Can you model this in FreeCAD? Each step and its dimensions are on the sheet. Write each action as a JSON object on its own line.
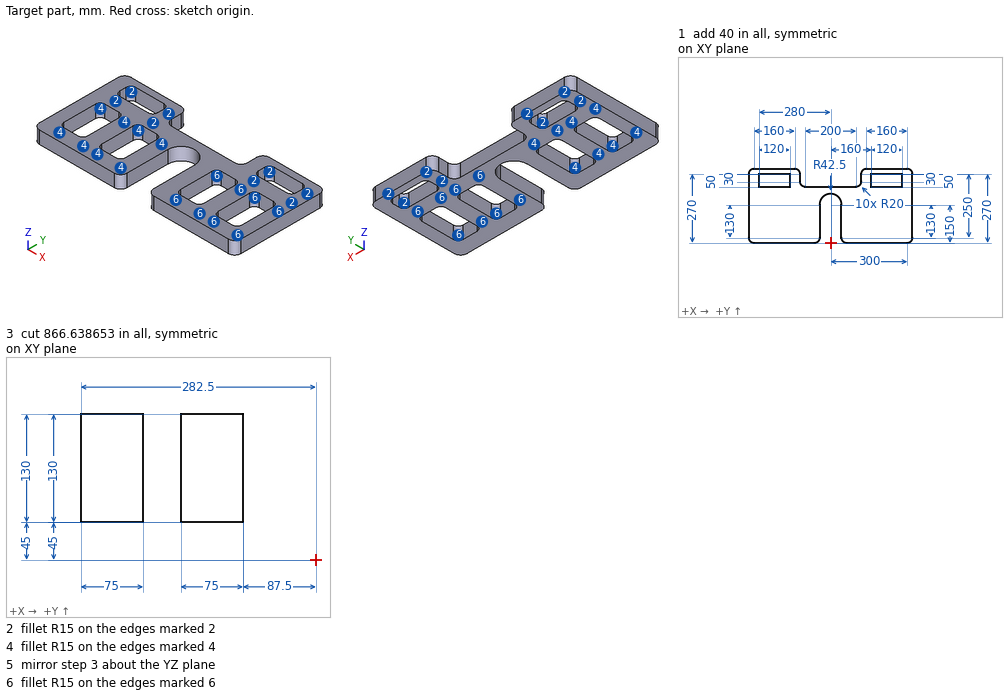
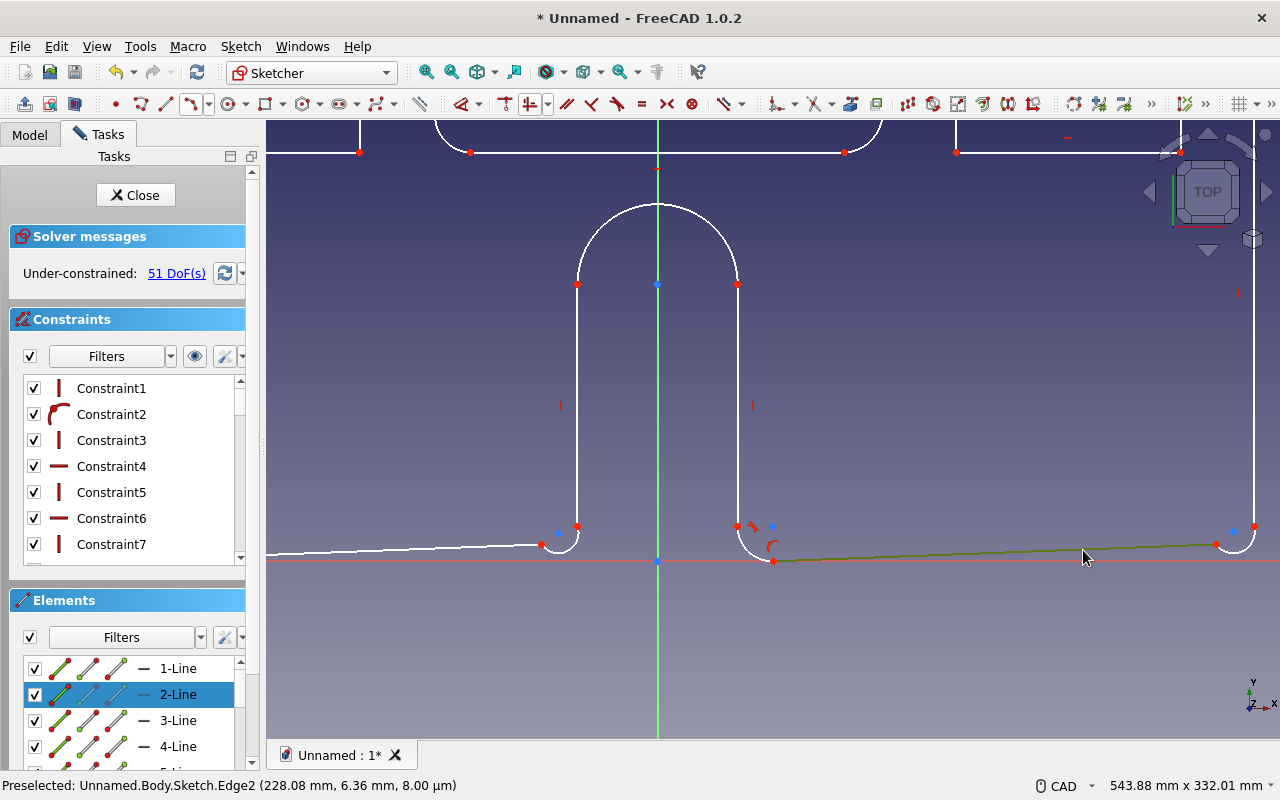
{"action": "left_click", "coordinate": [742, 543]}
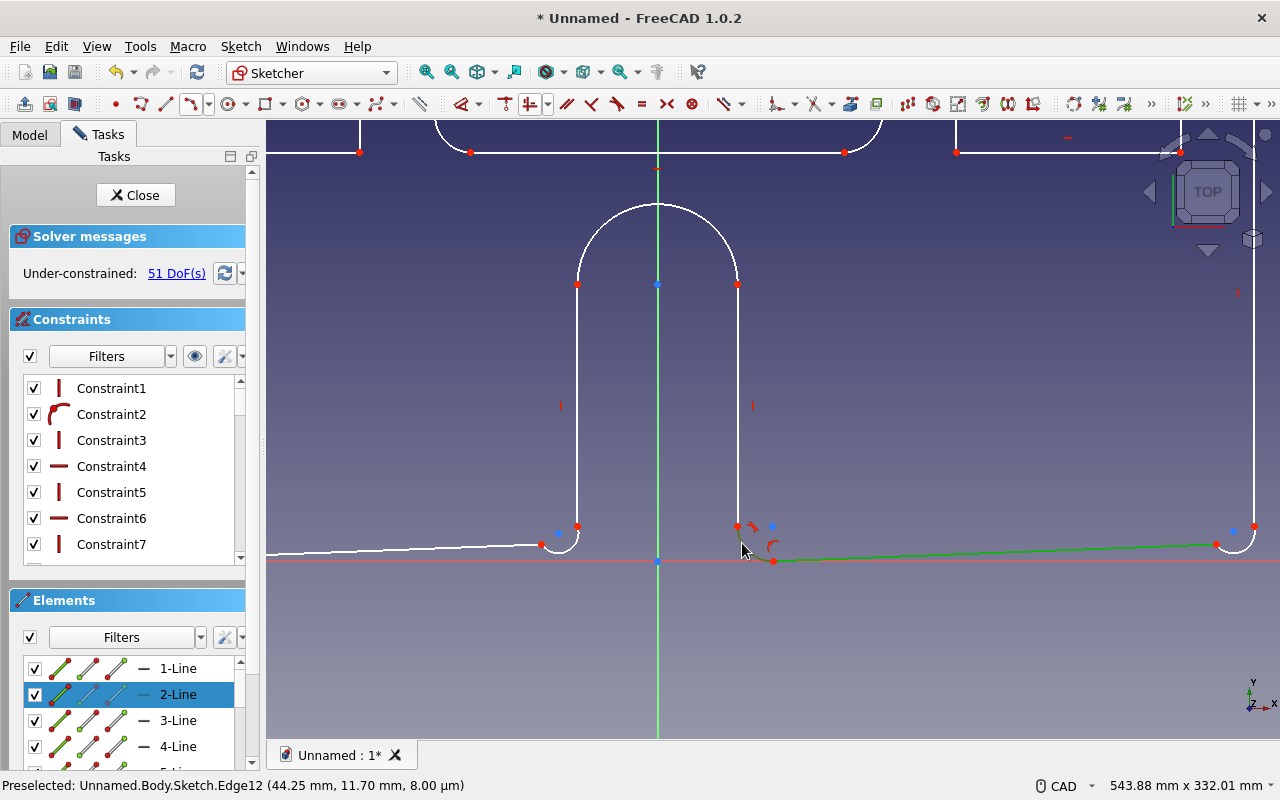
{"action": "left_click", "coordinate": [617, 104]}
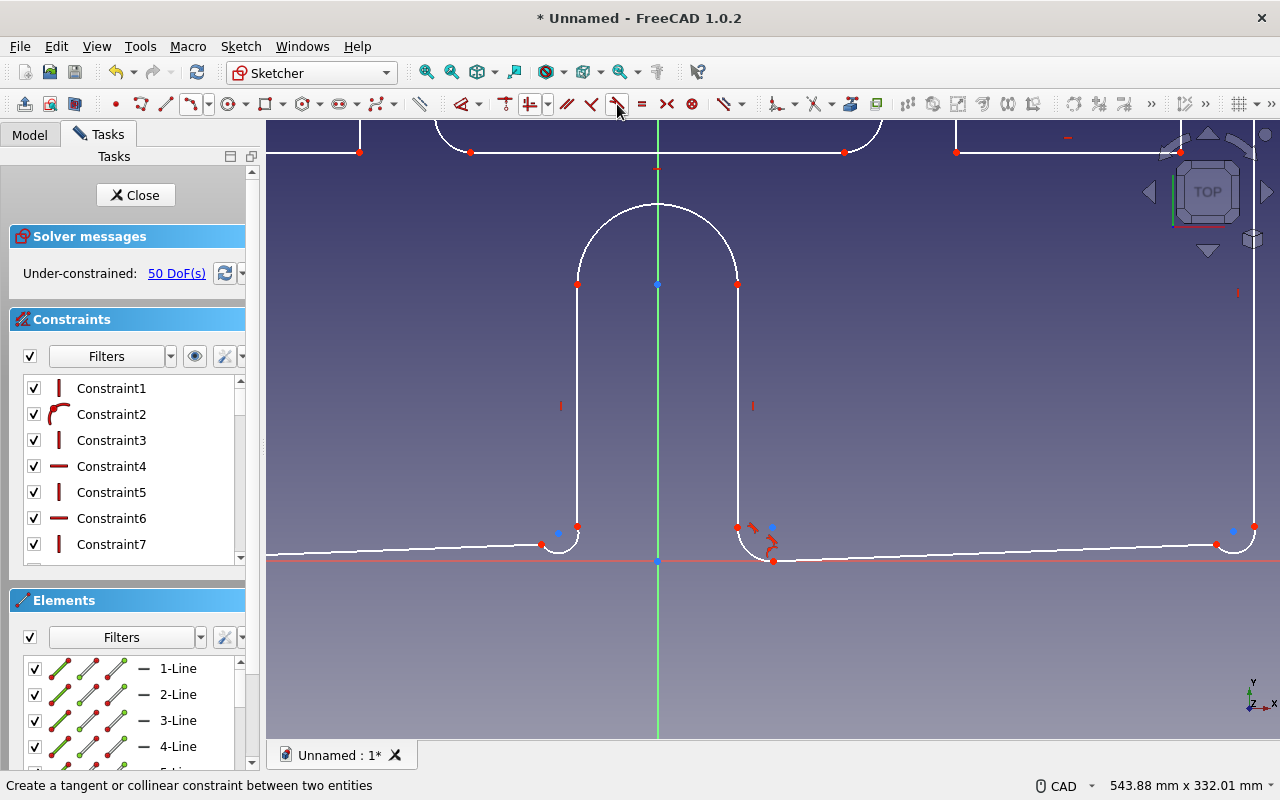
{"action": "left_click", "coordinate": [1083, 550]}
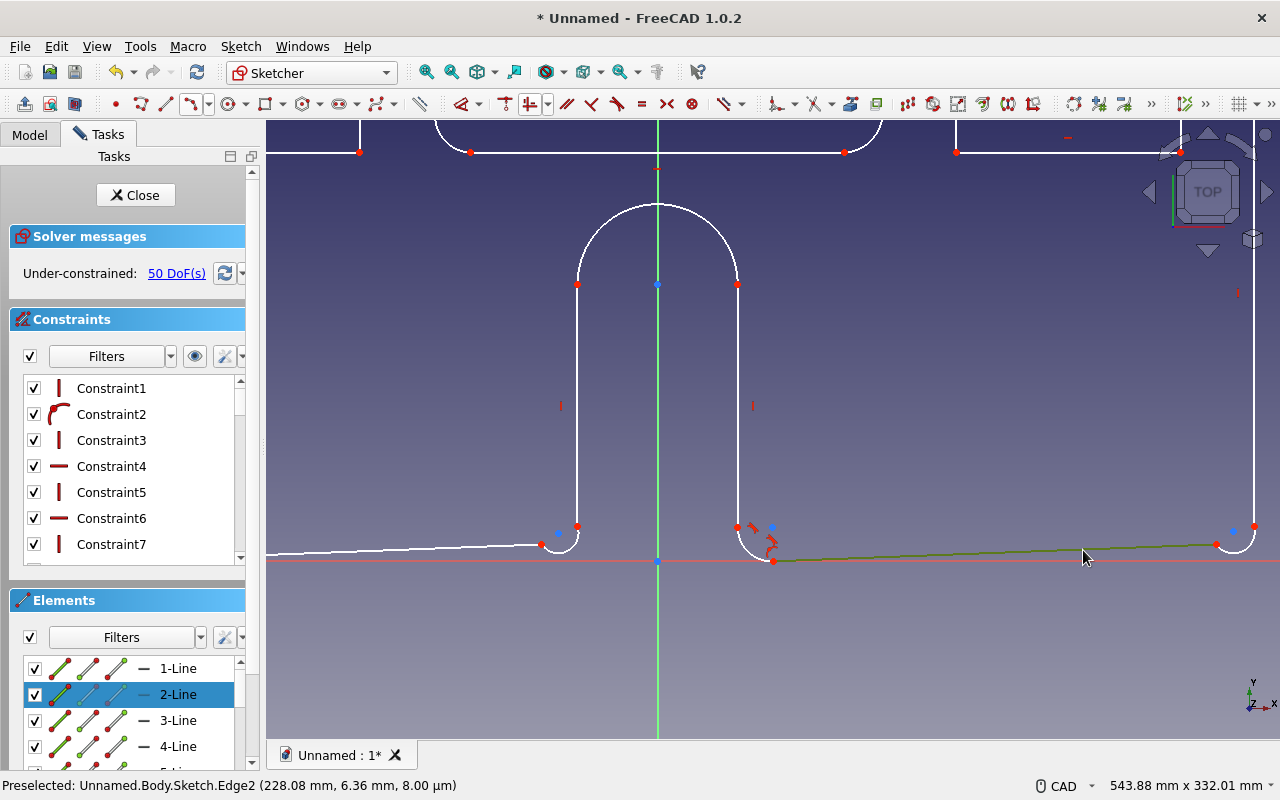
{"action": "scroll", "coordinate": [743, 542], "scroll_direction": "down", "scroll_amount": 4}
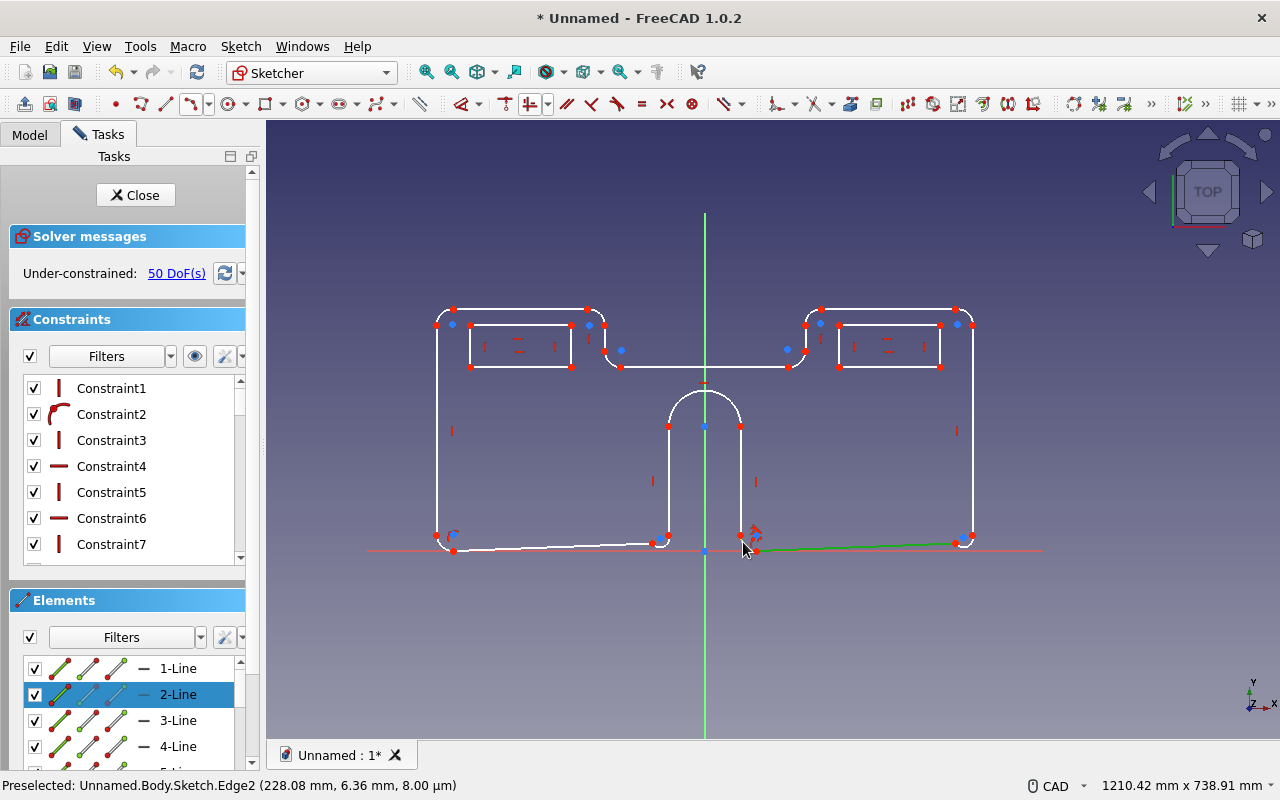
{"action": "scroll", "coordinate": [972, 543], "scroll_direction": "up", "scroll_amount": 3}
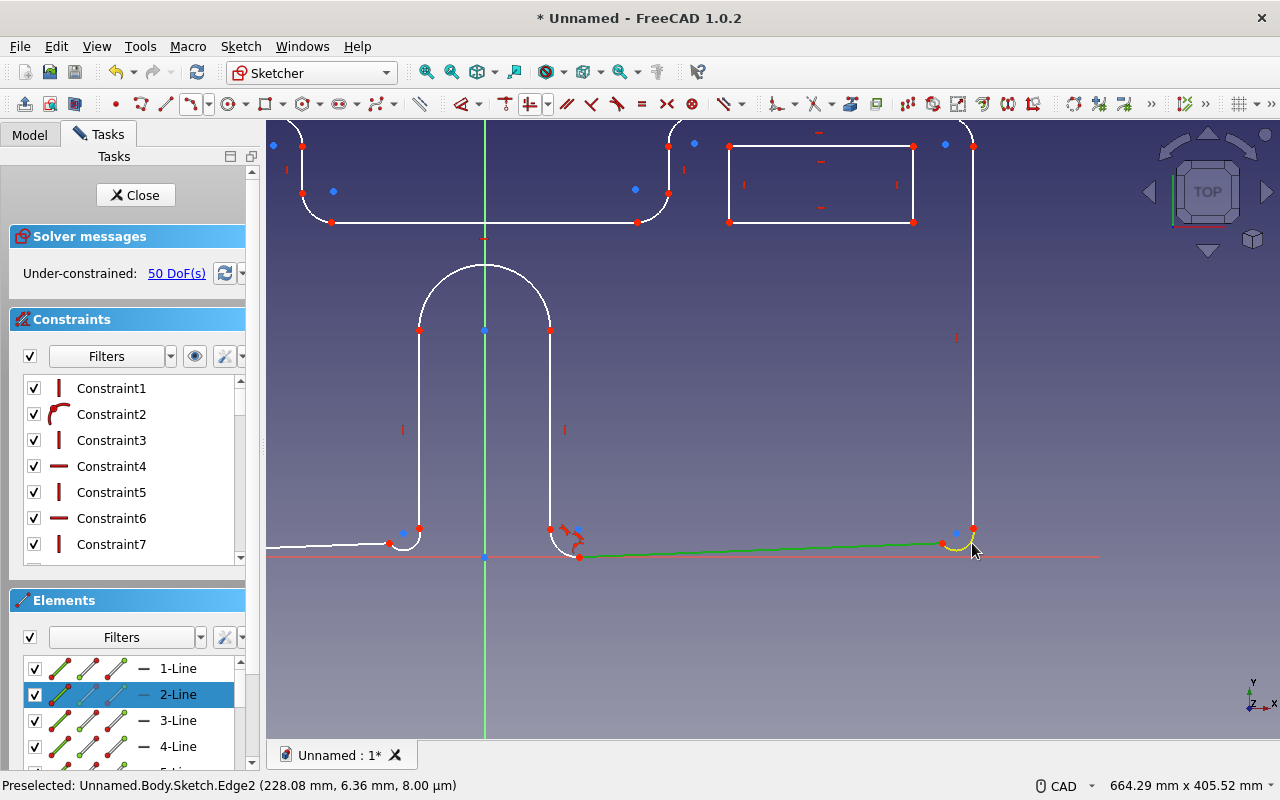
{"action": "left_click", "coordinate": [971, 543]}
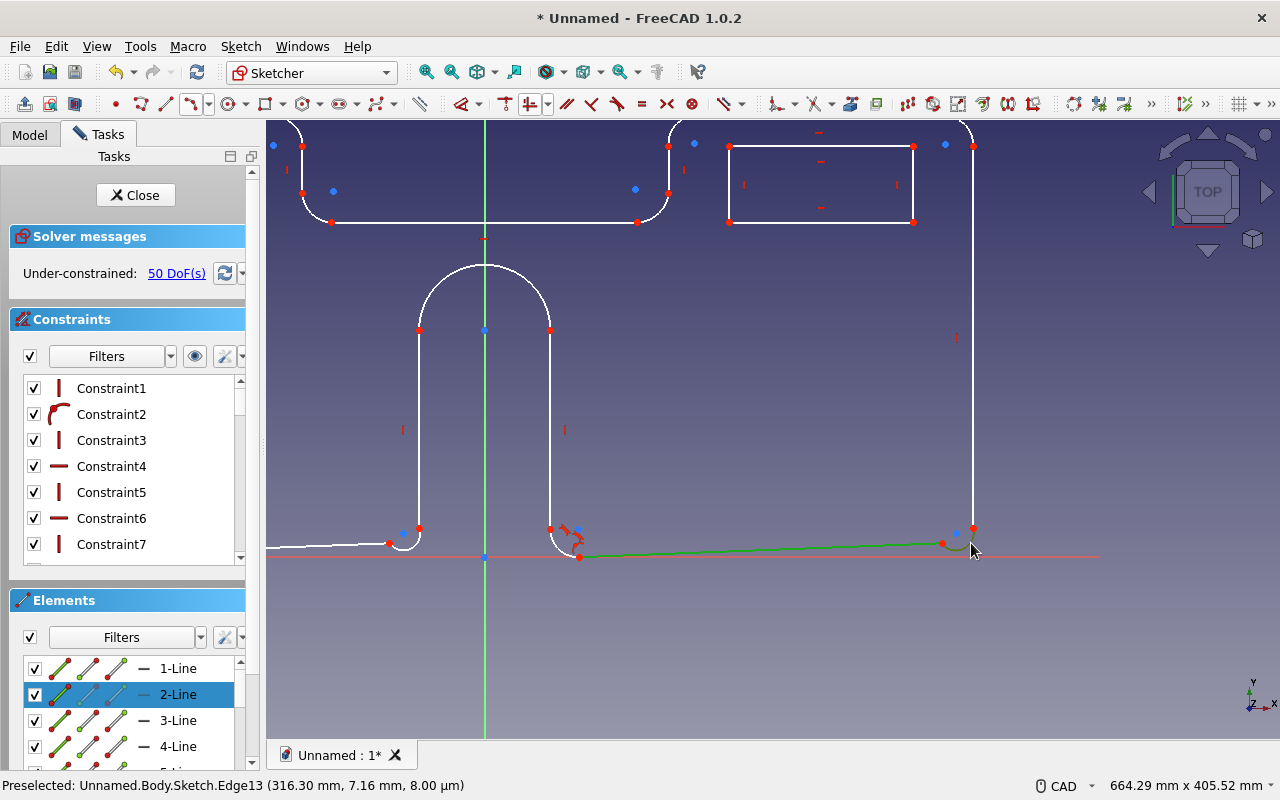
{"action": "key", "text": "t"}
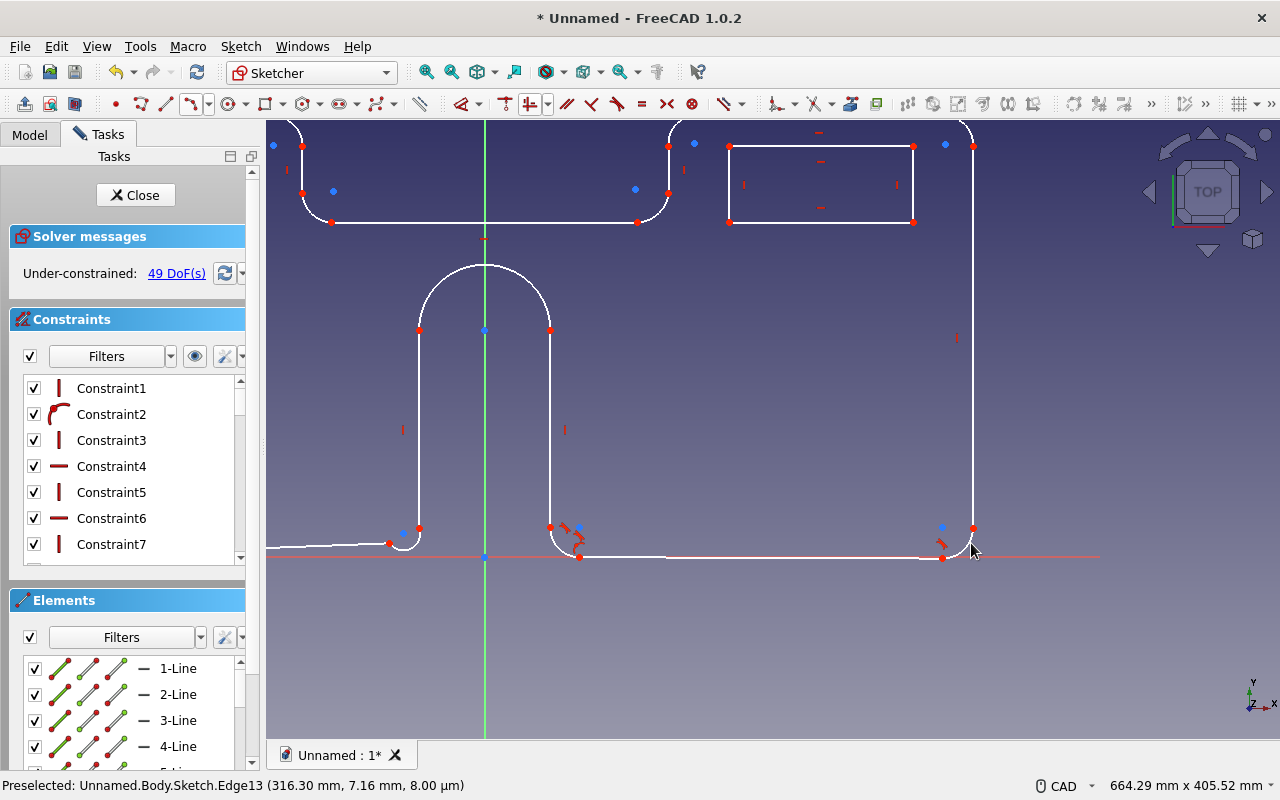
{"action": "left_click", "coordinate": [973, 414]}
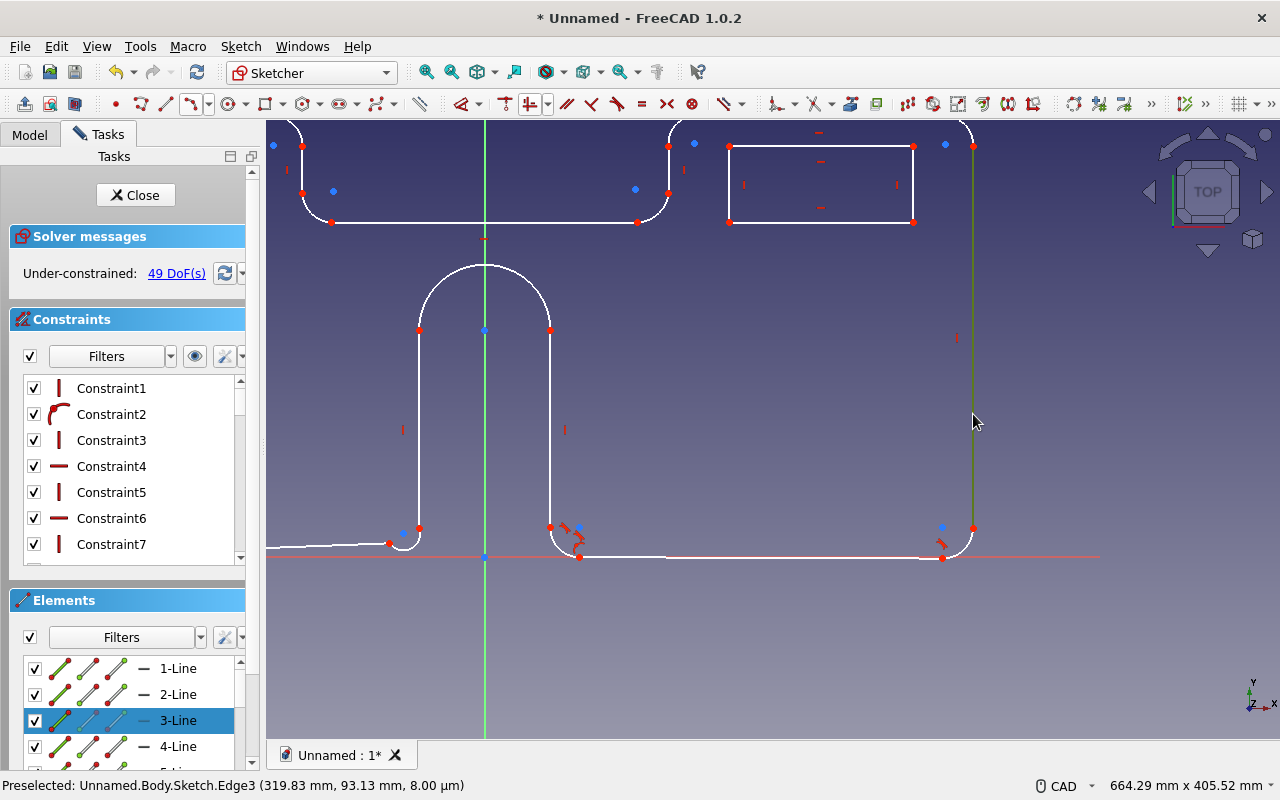
{"action": "left_click", "coordinate": [956, 555]}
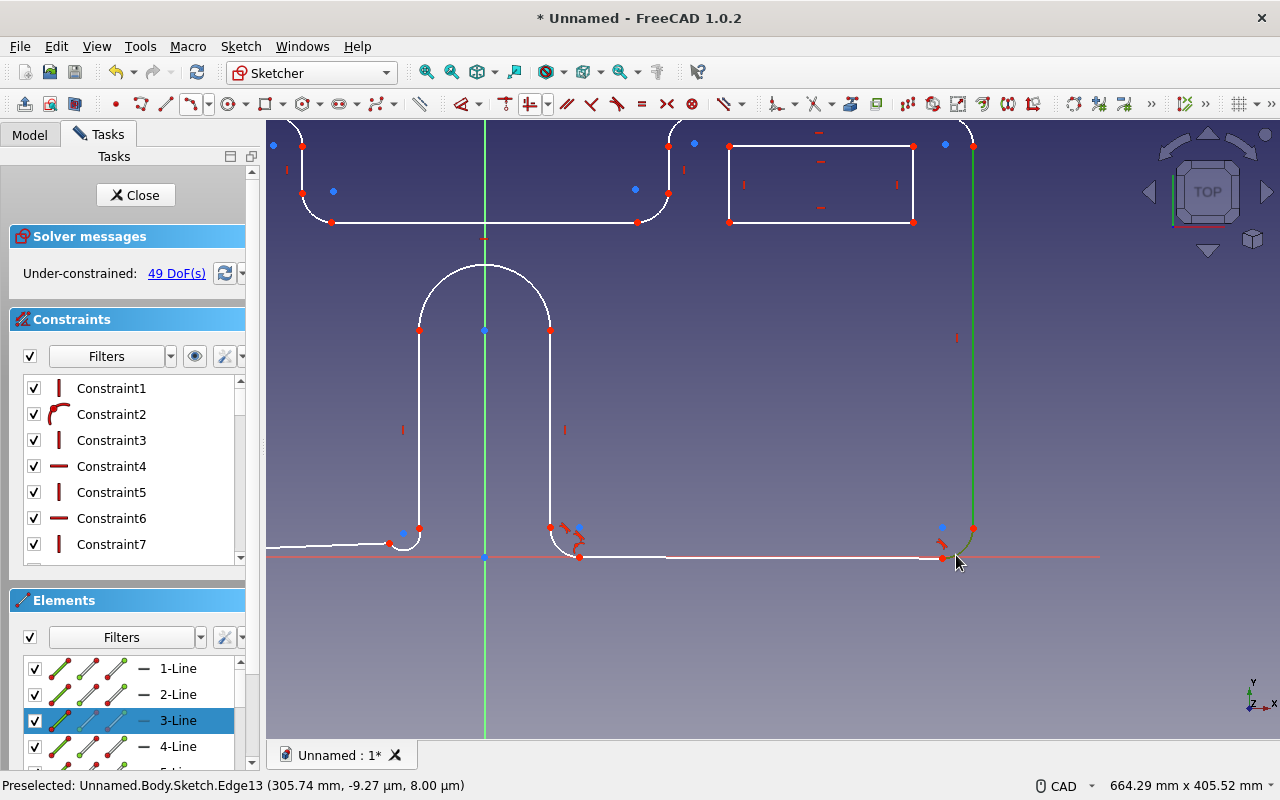
{"action": "left_click", "coordinate": [617, 104]}